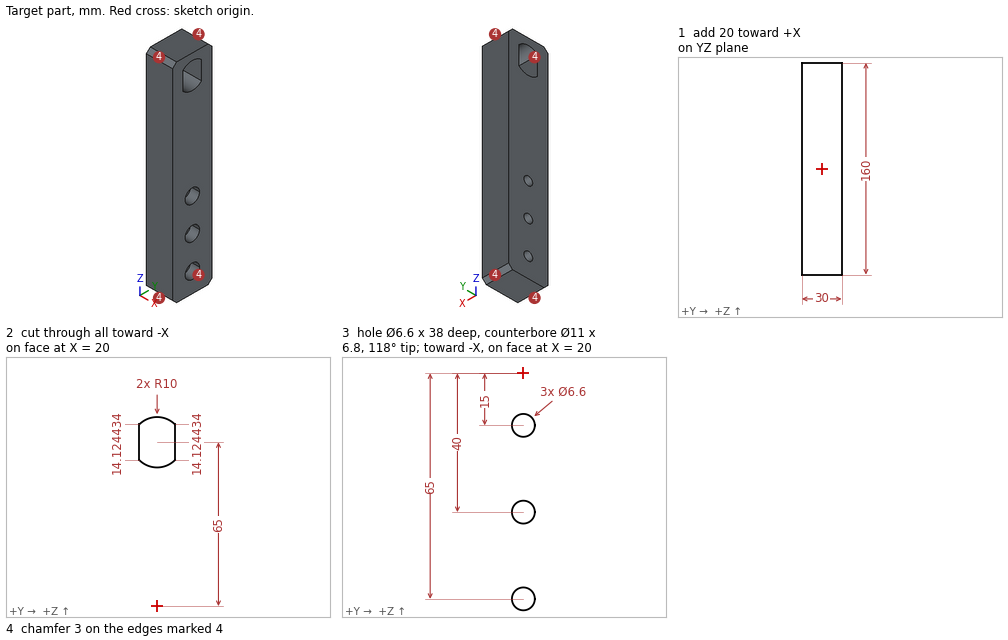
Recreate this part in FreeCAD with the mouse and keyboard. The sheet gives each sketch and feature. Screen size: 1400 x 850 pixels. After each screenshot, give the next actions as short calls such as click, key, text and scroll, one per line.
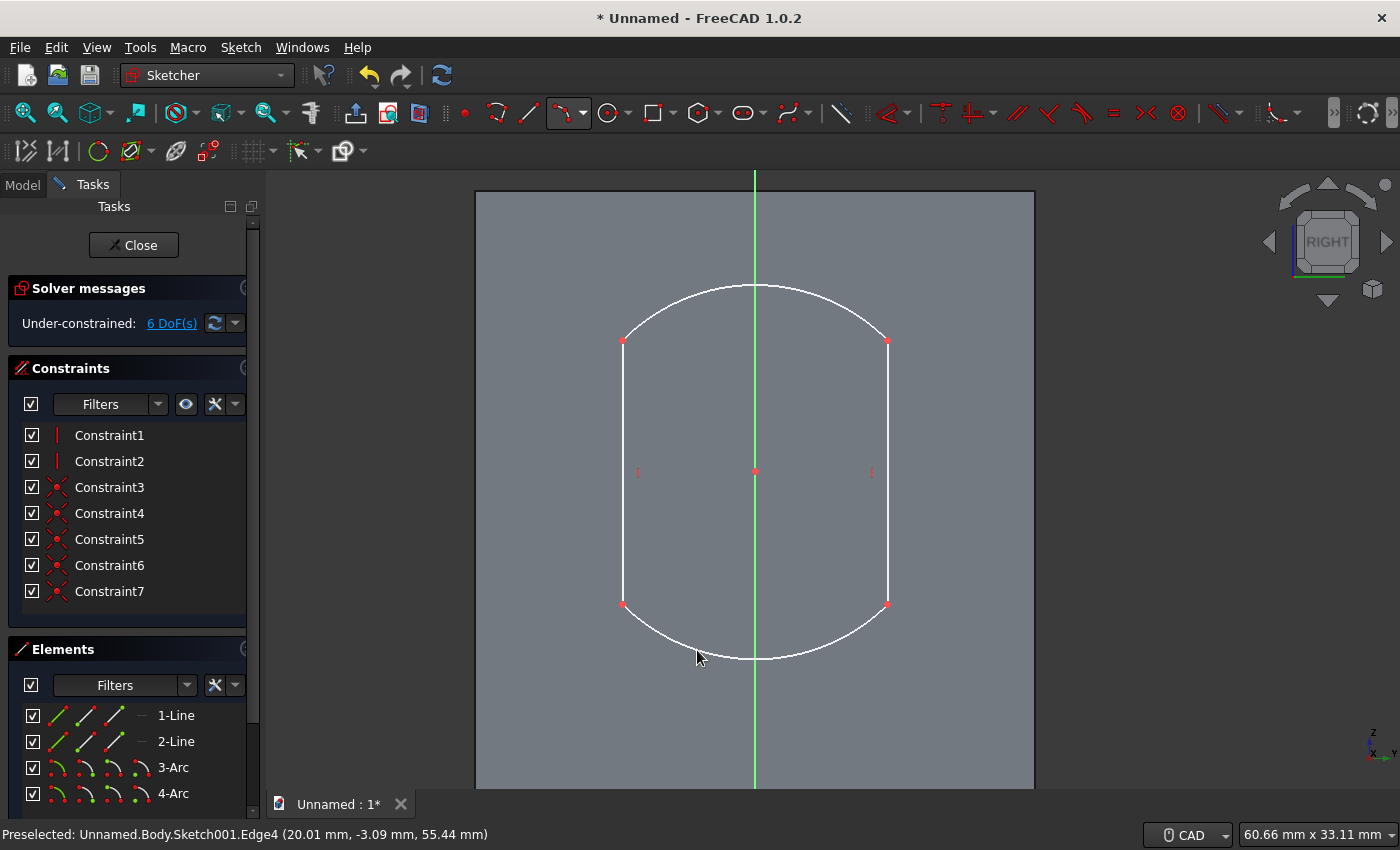
click(813, 294)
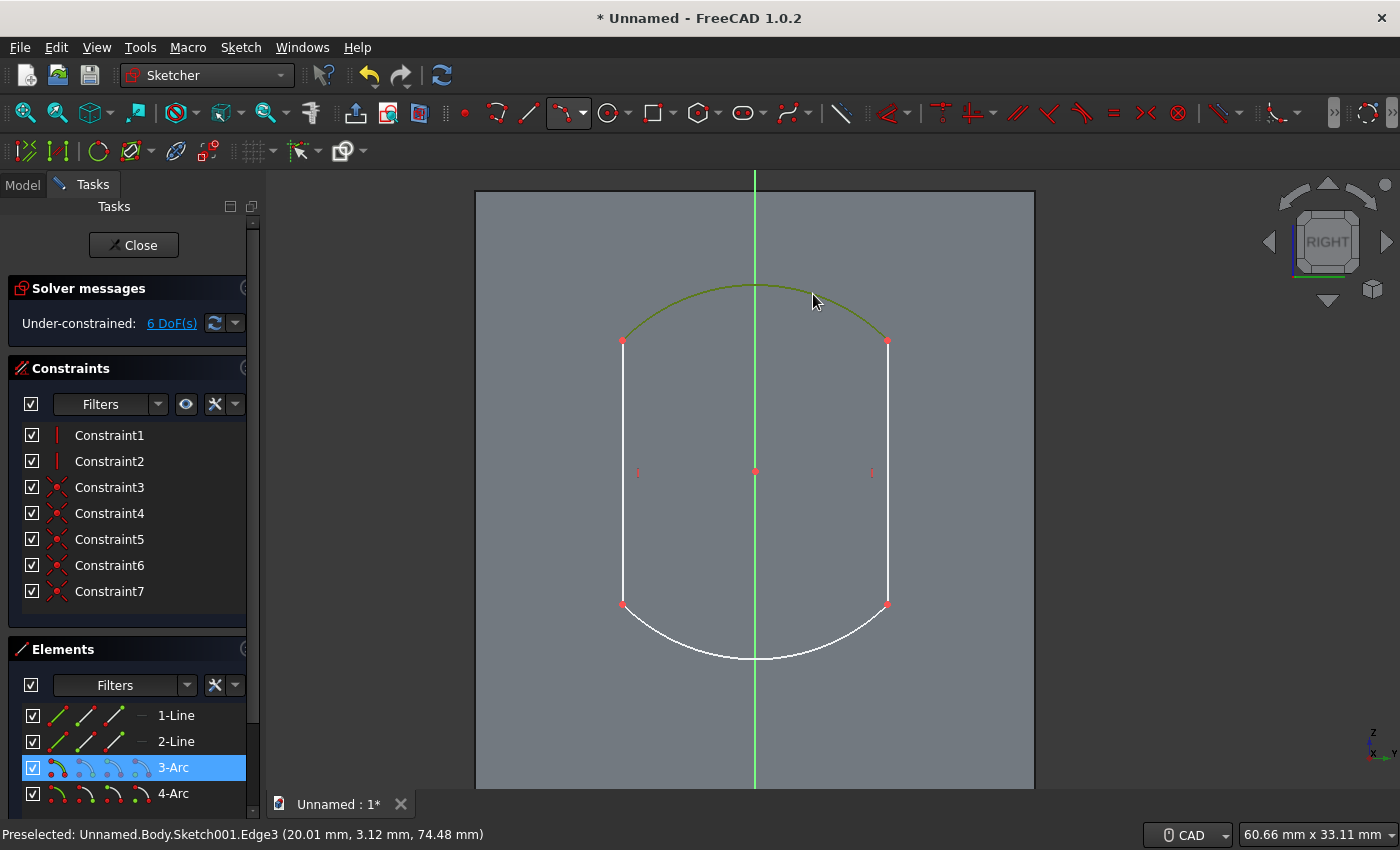
click(697, 650)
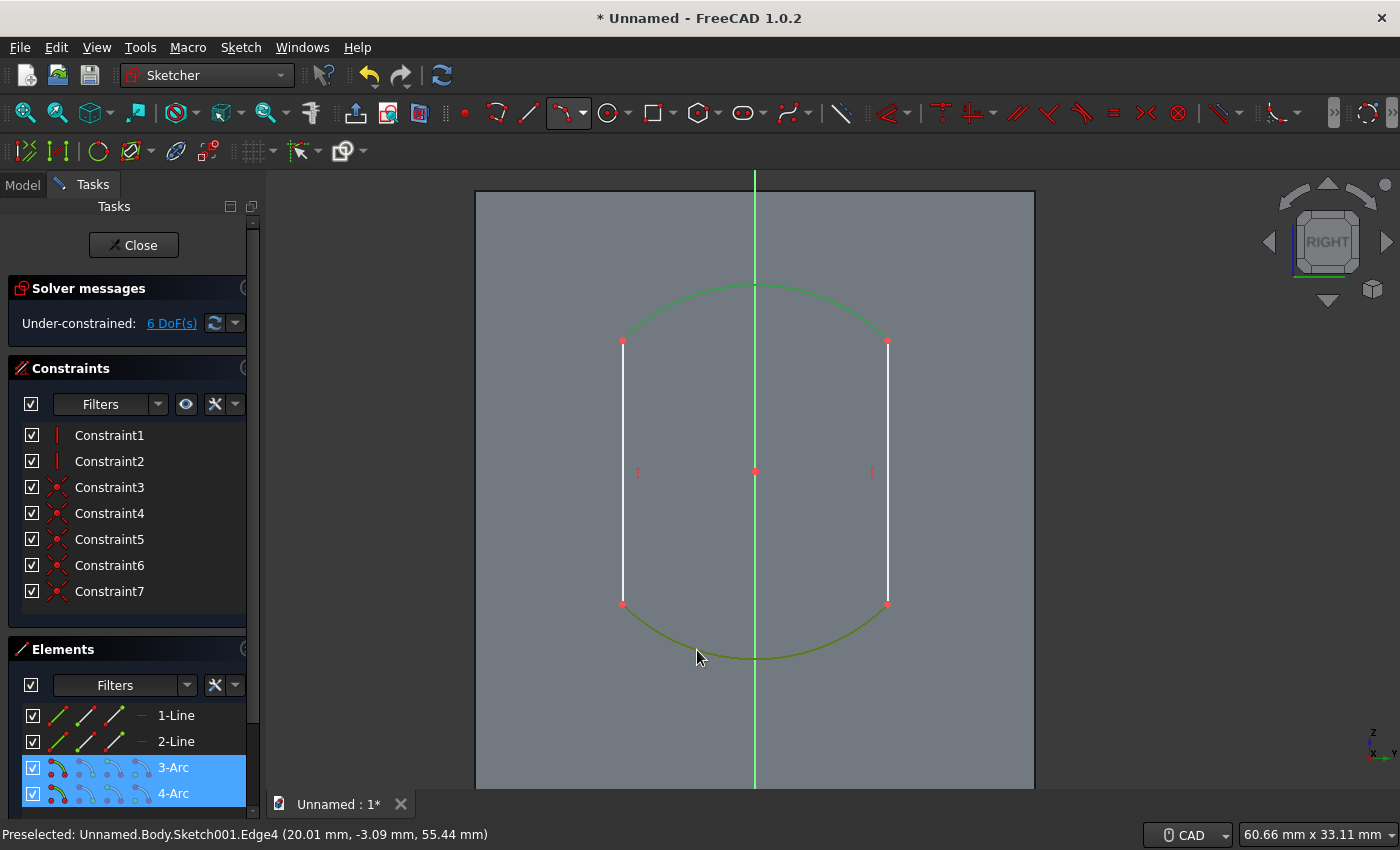
click(1114, 114)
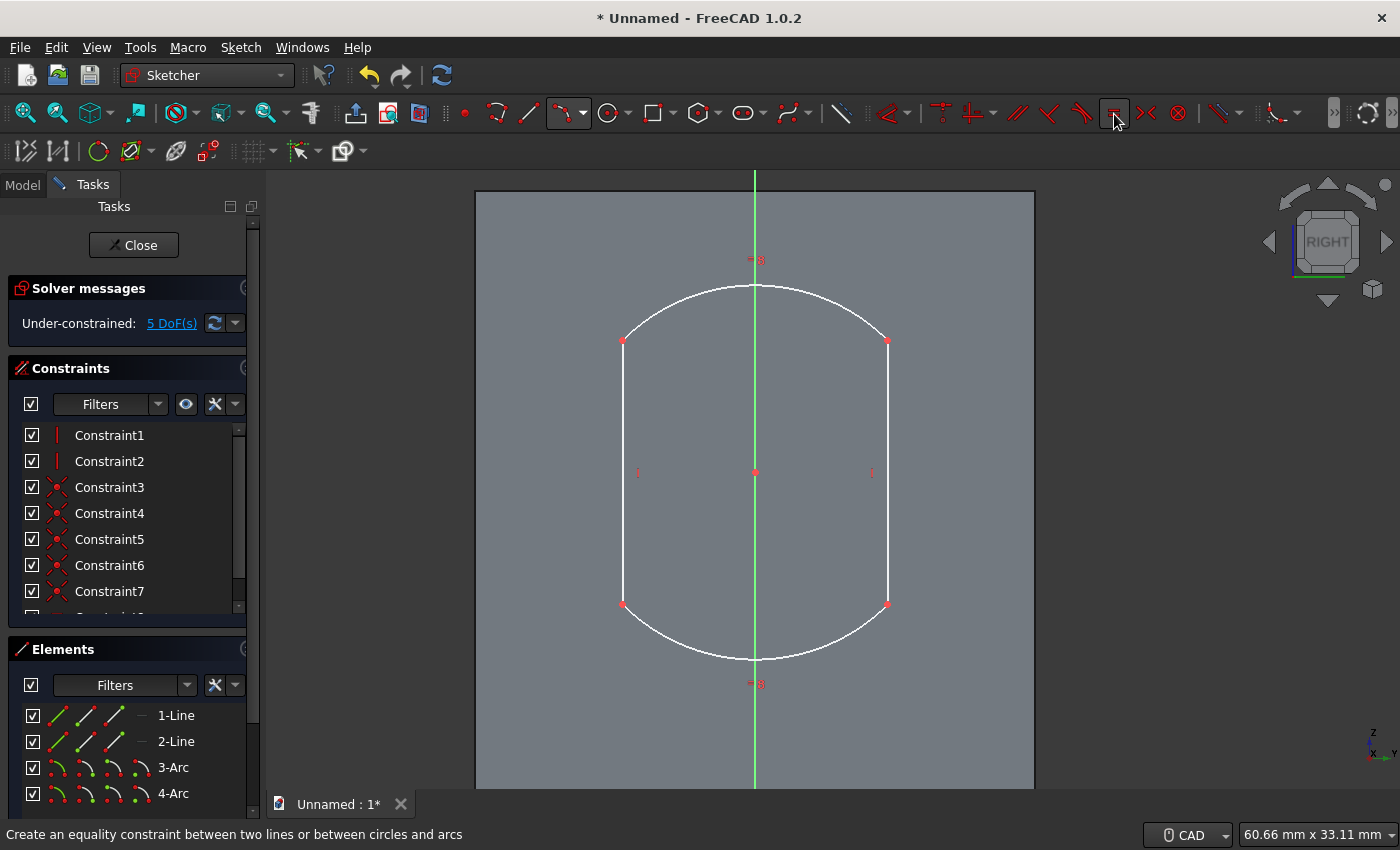
click(755, 473)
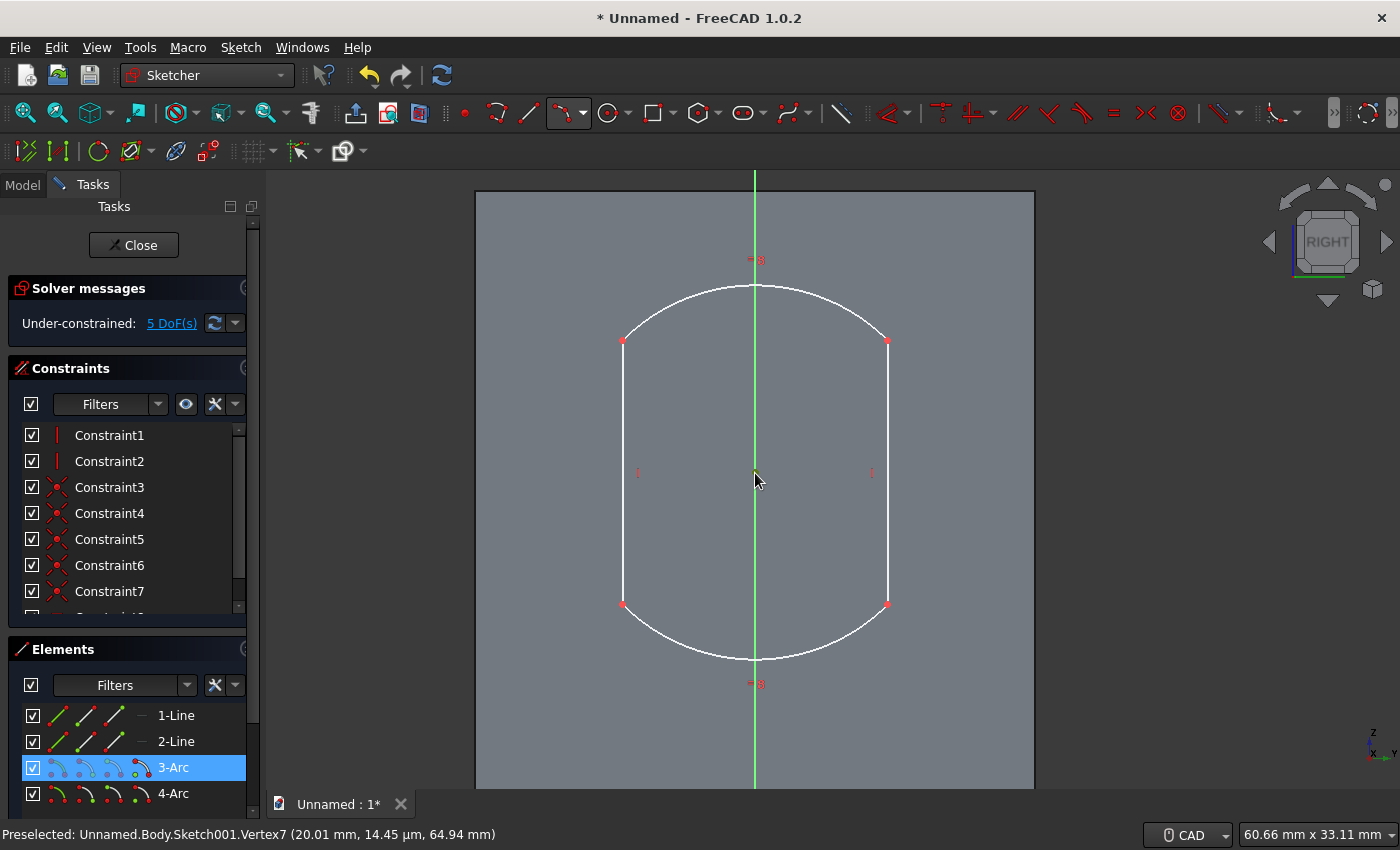
click(755, 721)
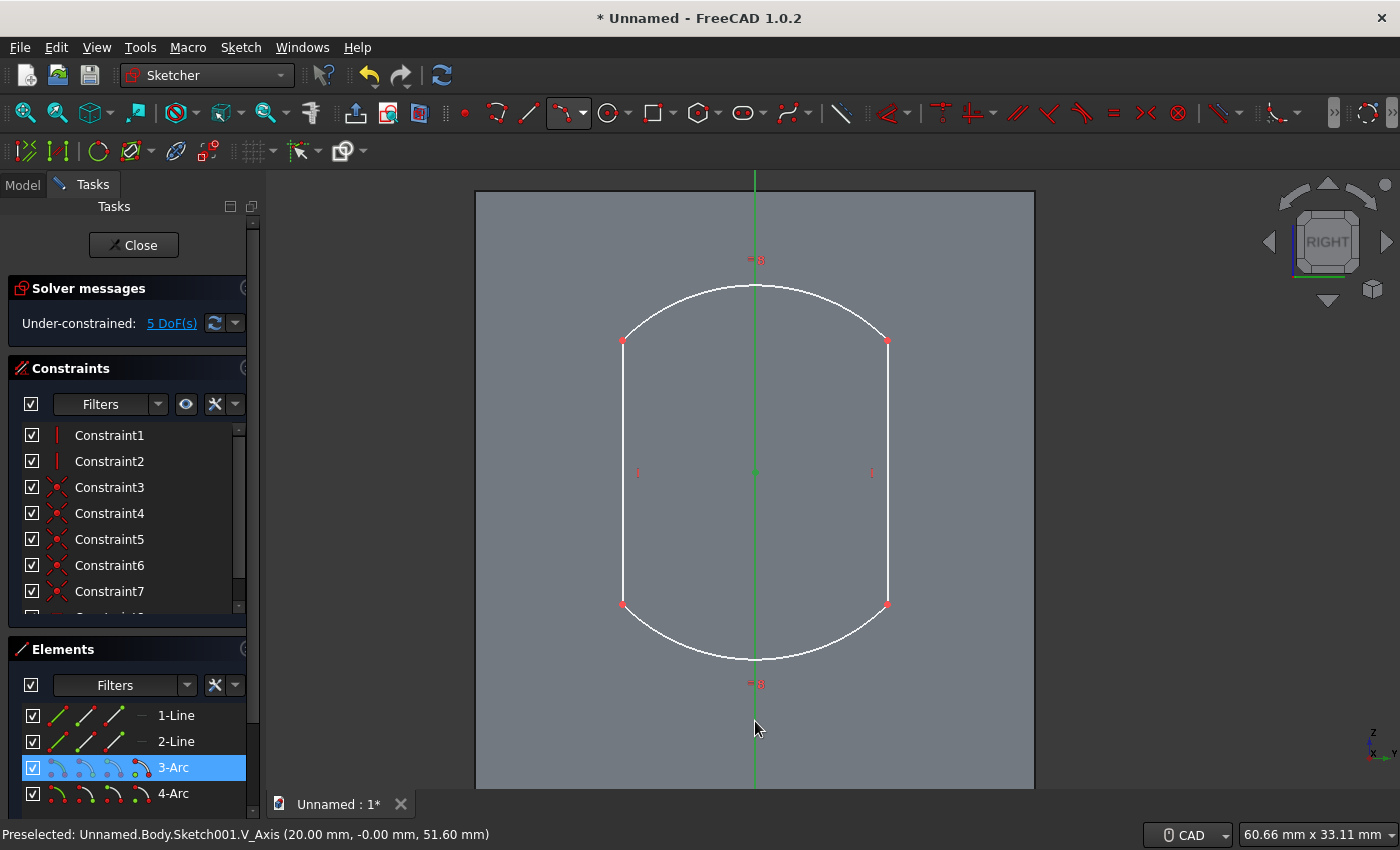
key(c)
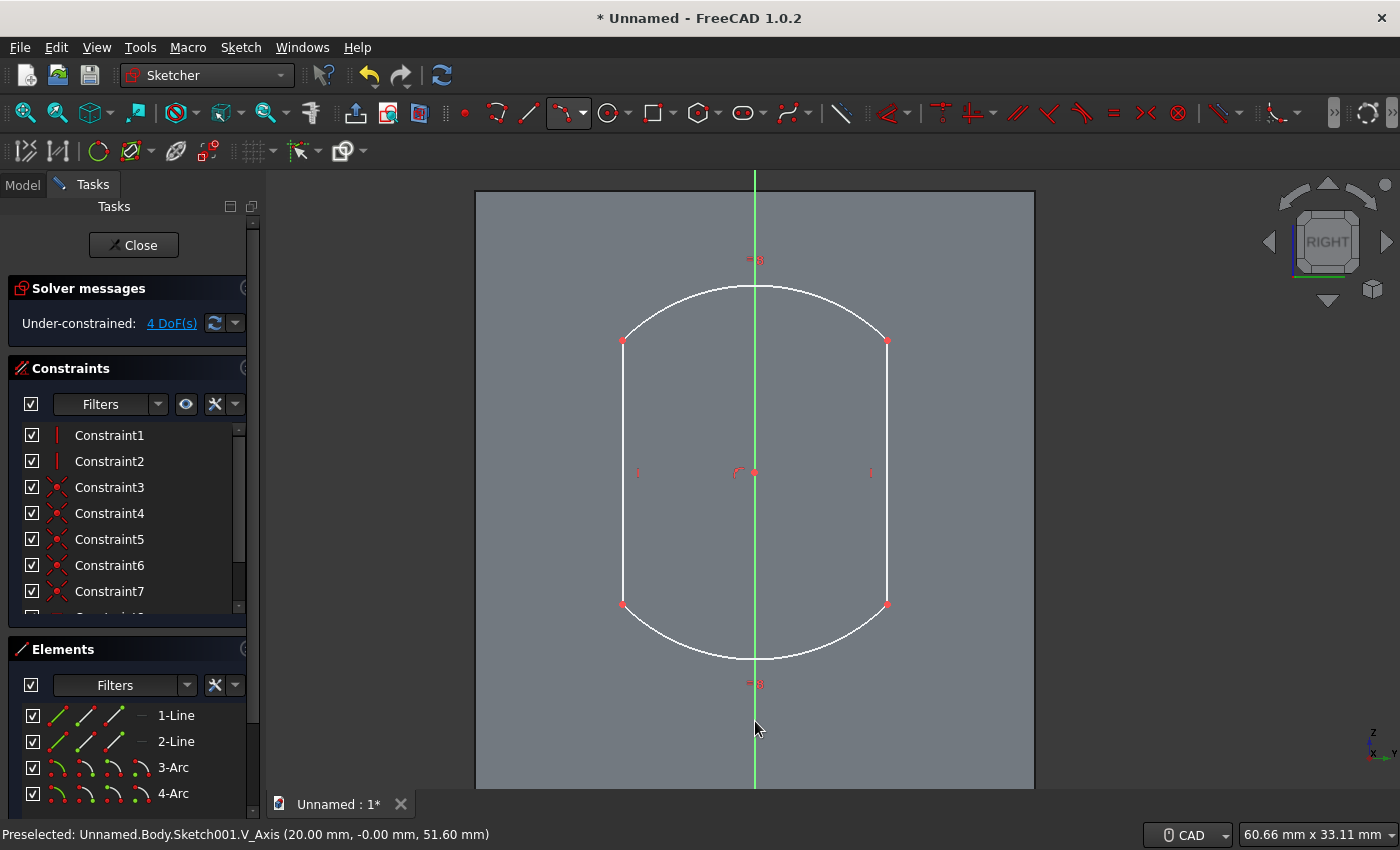
key(d)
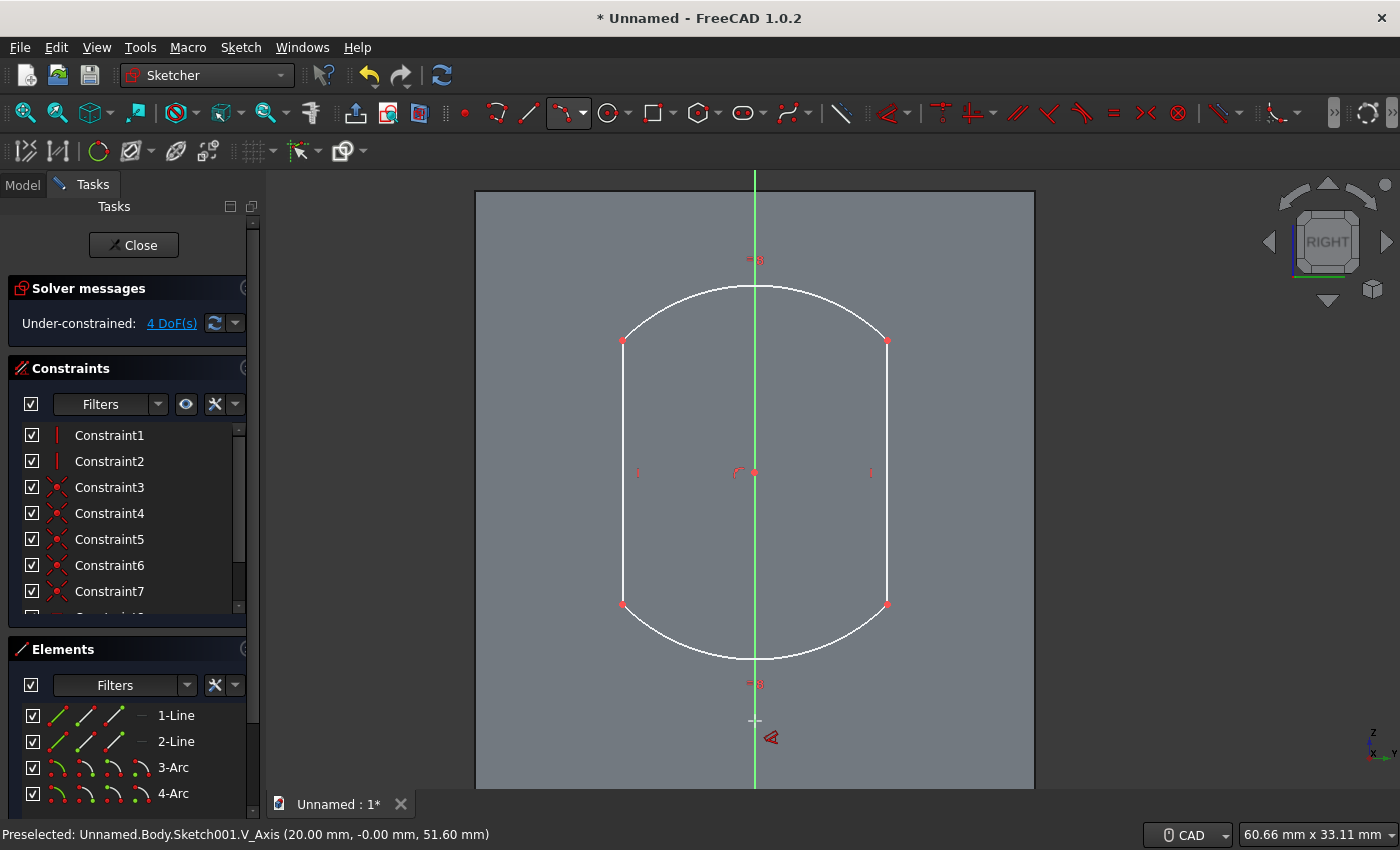
click(813, 295)
click(823, 265)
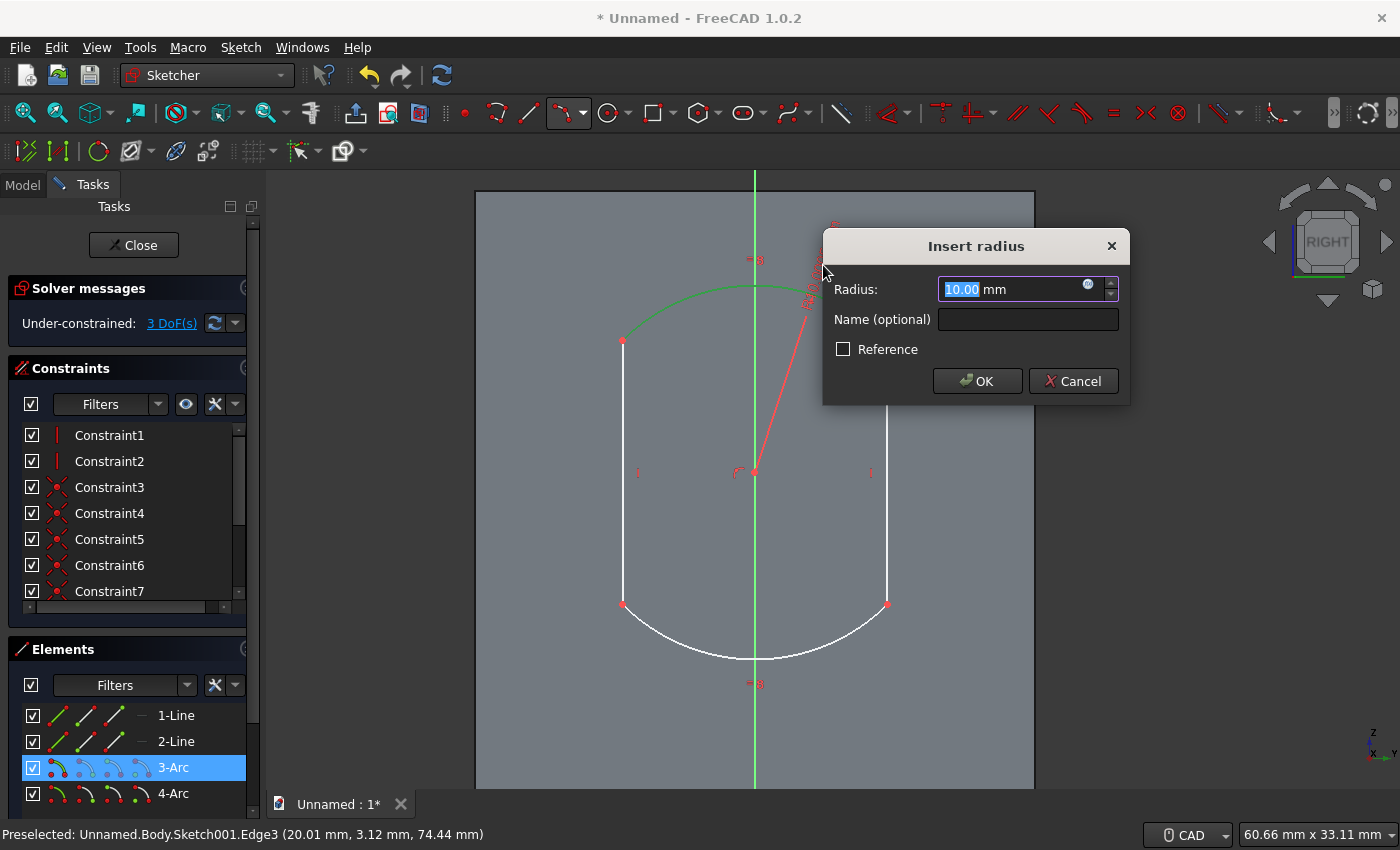
text(10)
key(Return)